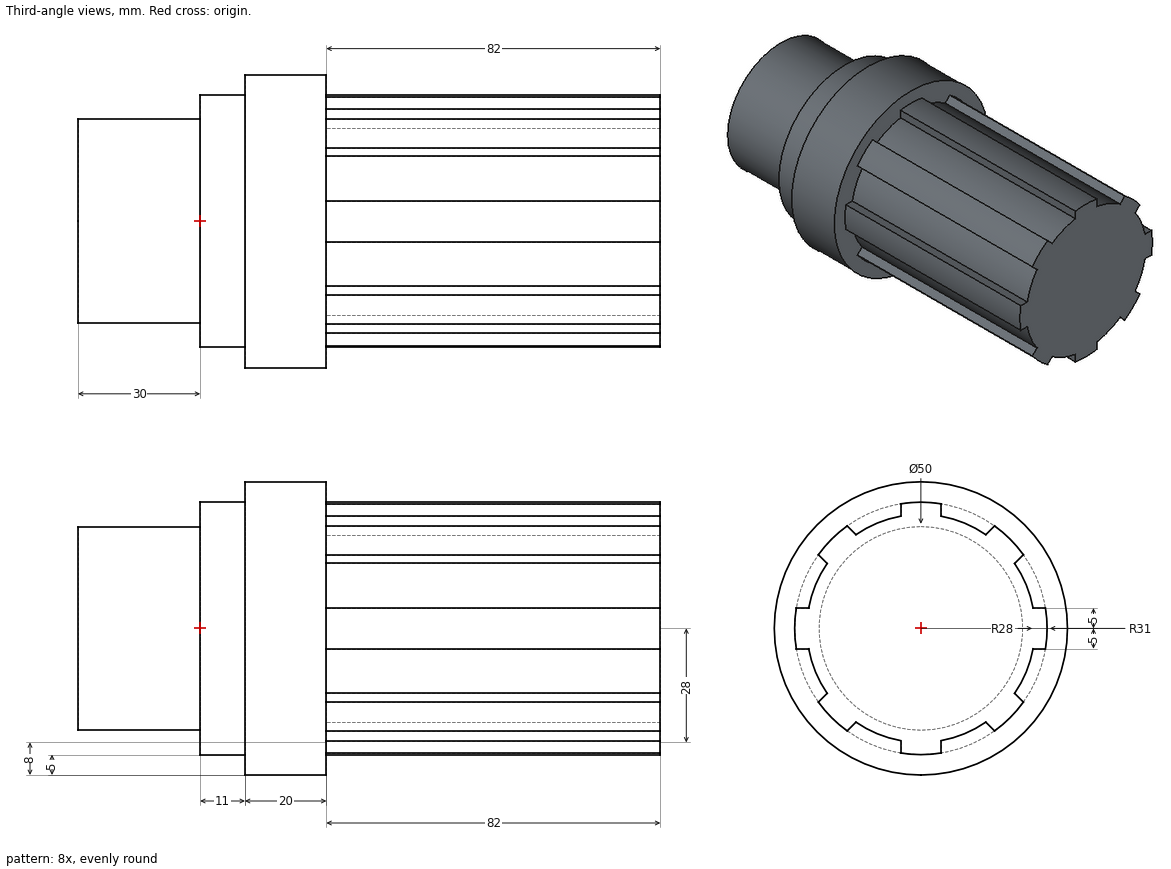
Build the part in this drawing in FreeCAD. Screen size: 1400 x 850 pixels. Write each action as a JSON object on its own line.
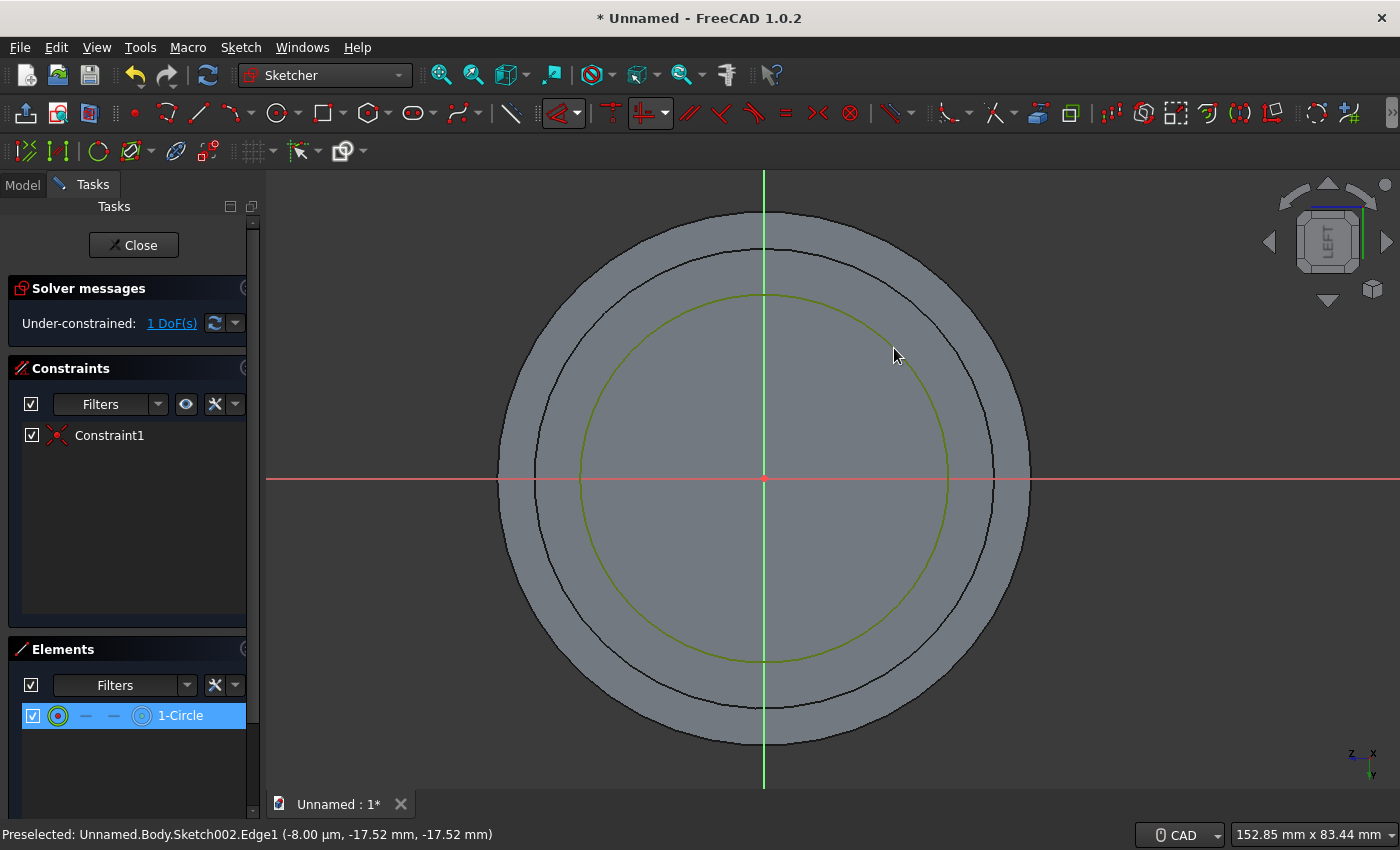
{"action": "key", "text": "k o"}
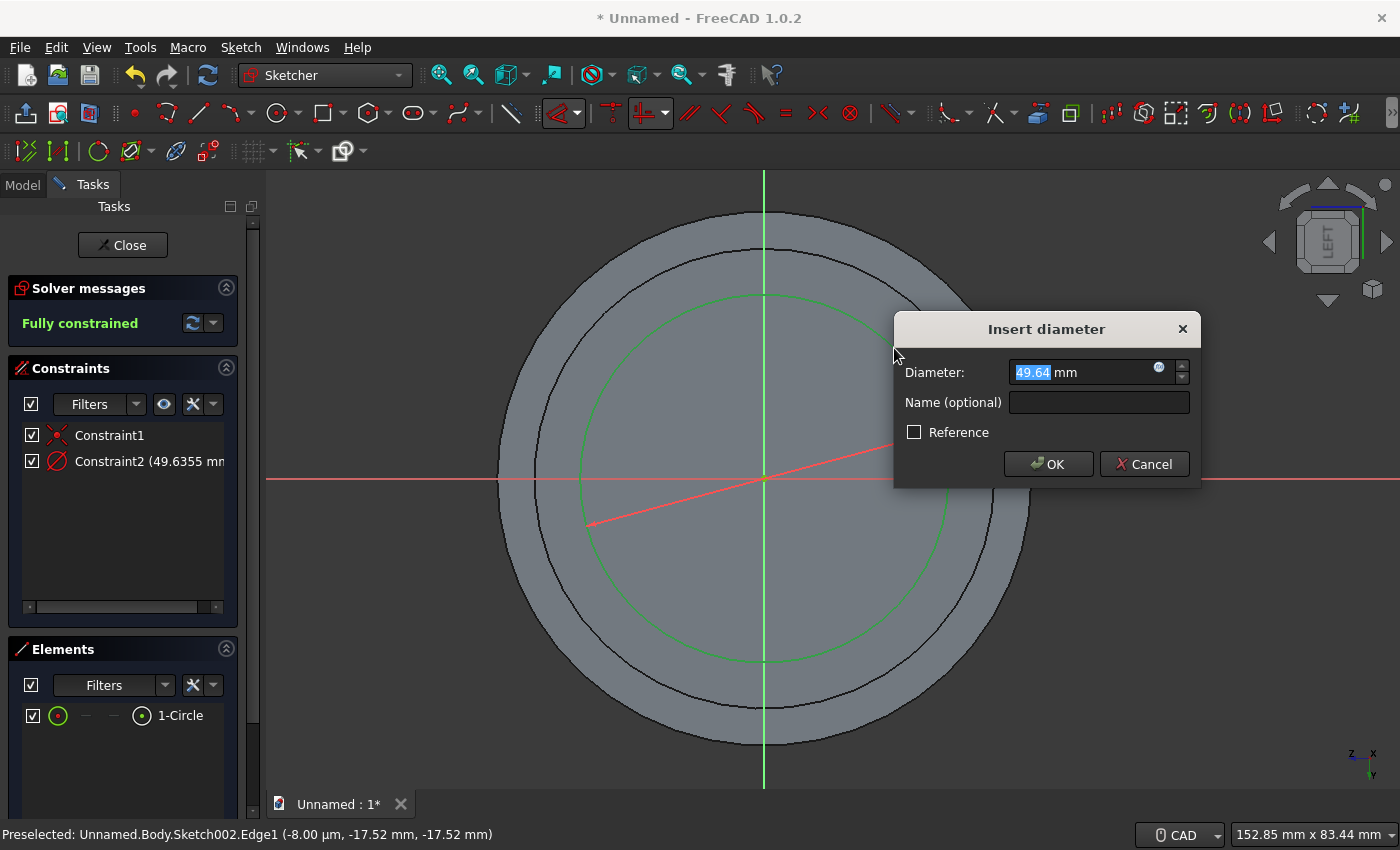
{"action": "type", "text": "50"}
{"action": "key", "text": "Return"}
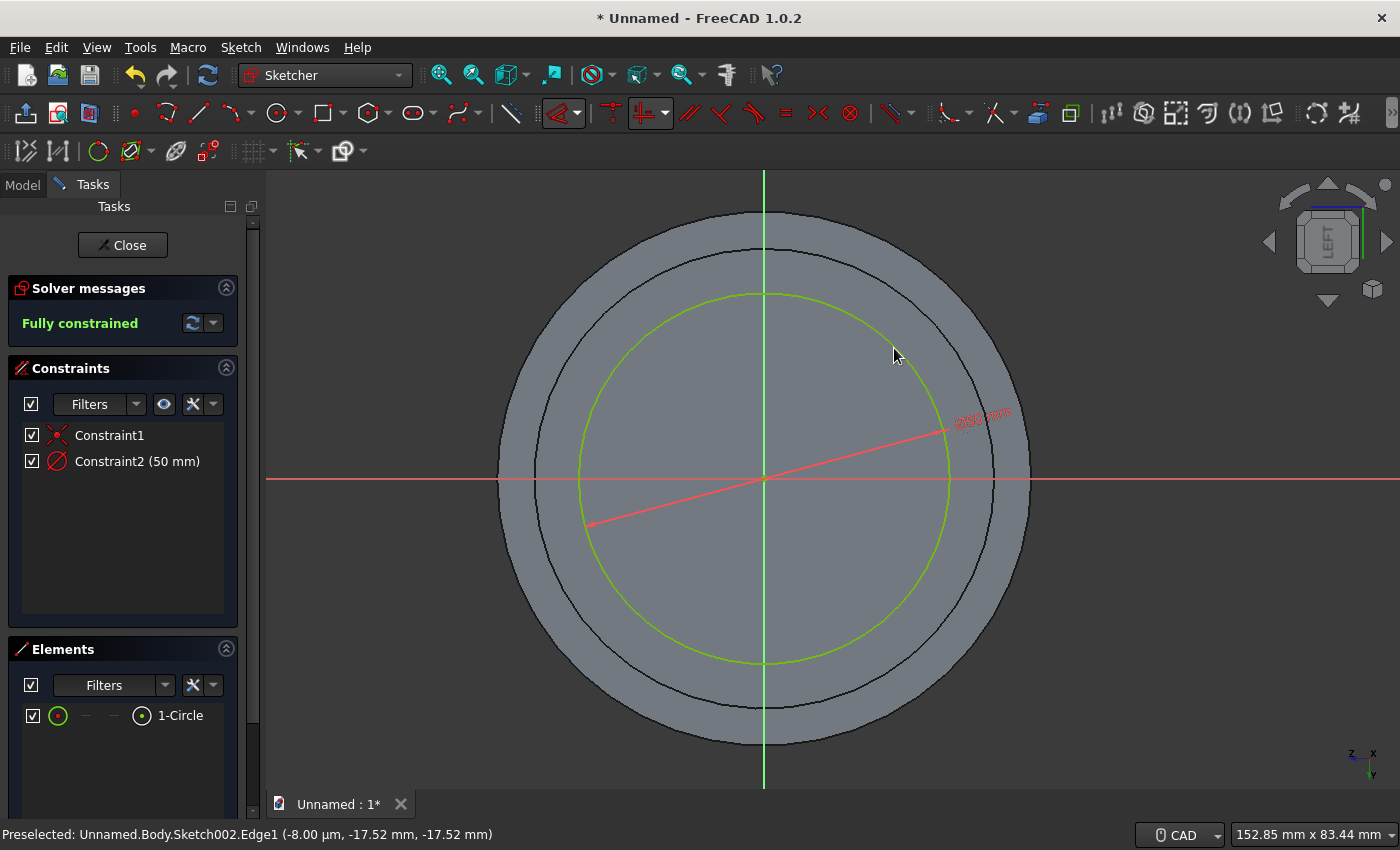
{"action": "left_click", "coordinate": [123, 245]}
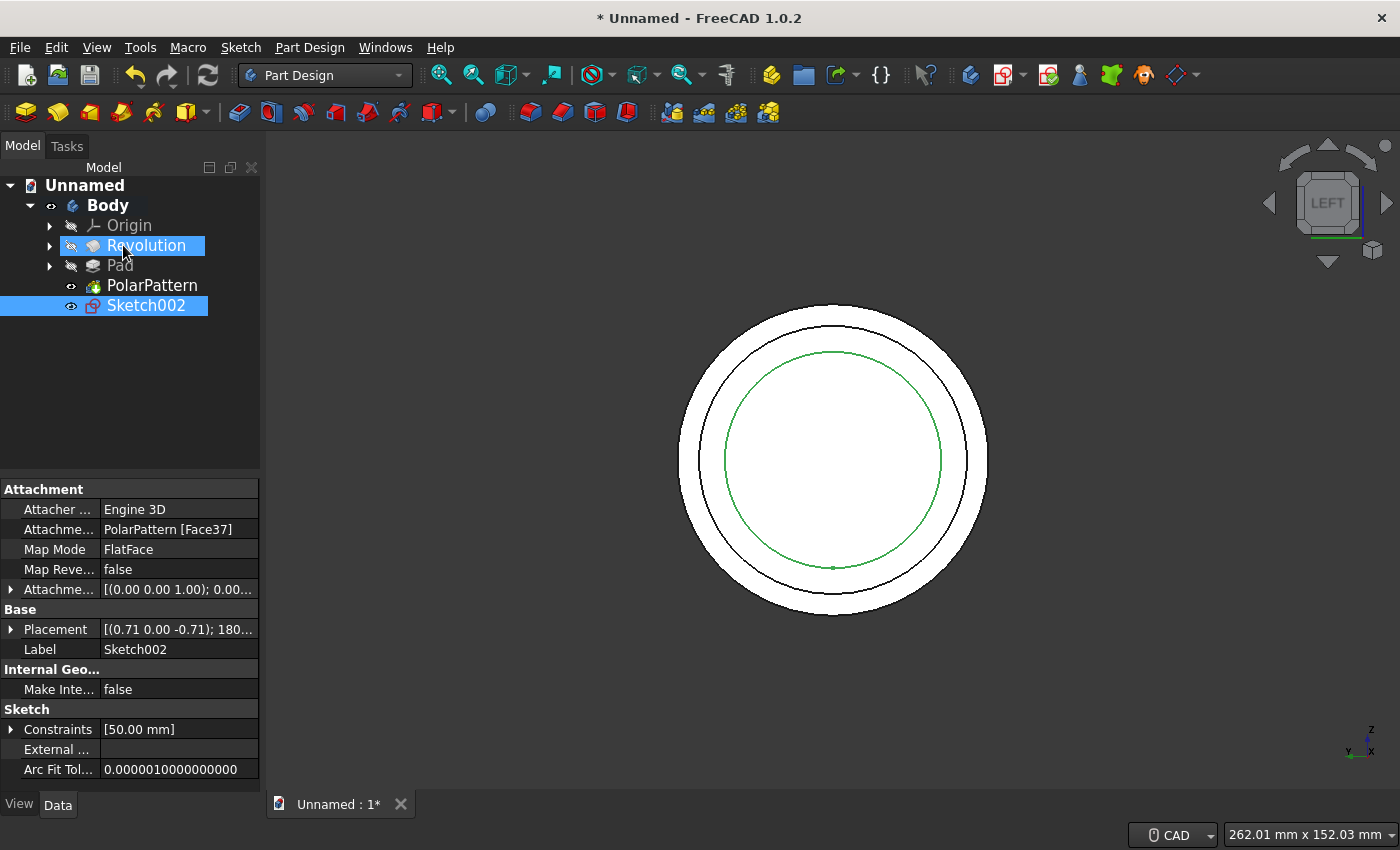
{"action": "left_click", "coordinate": [26, 112]}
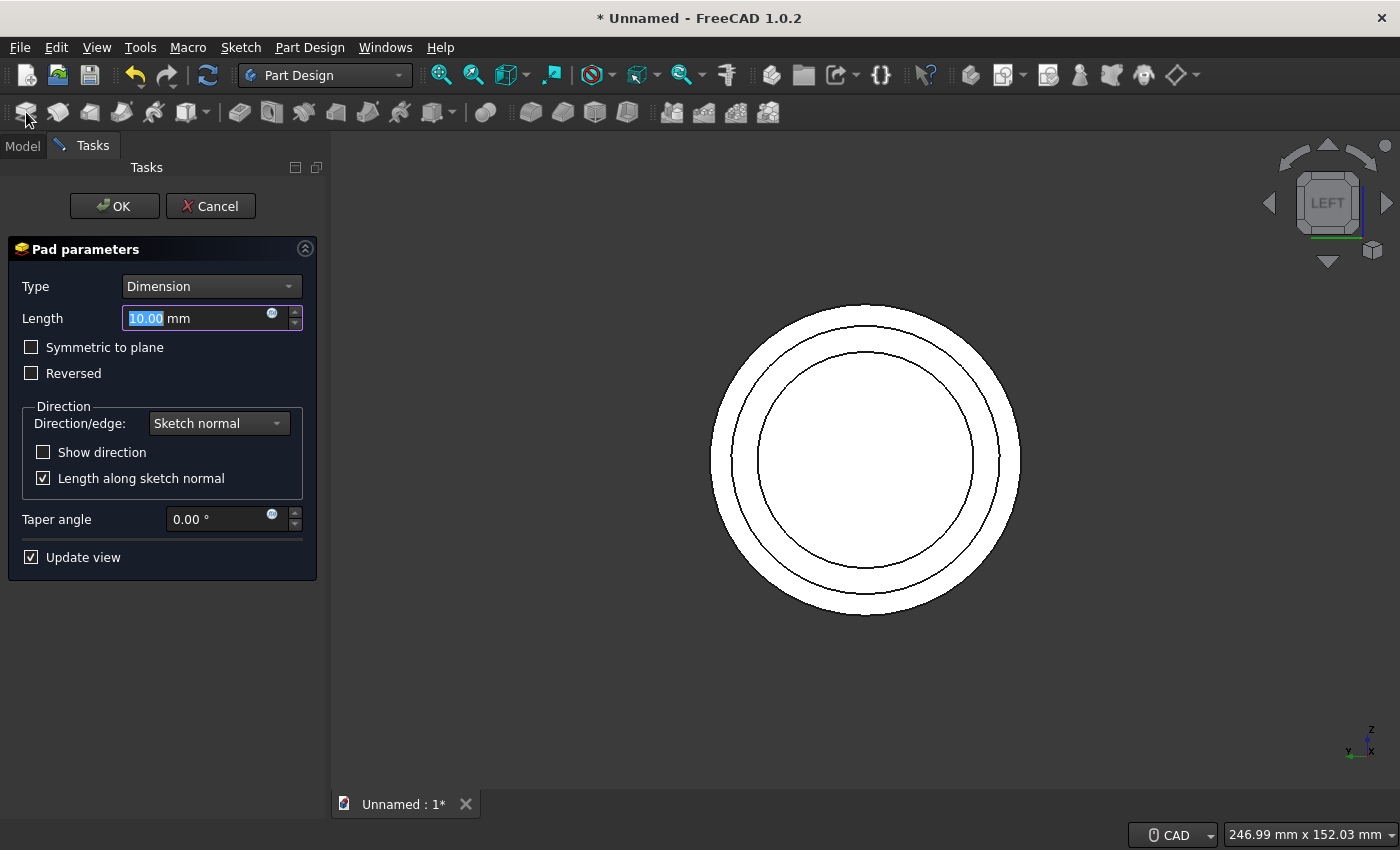
{"action": "type", "text": "30"}
{"action": "key", "text": "Tab"}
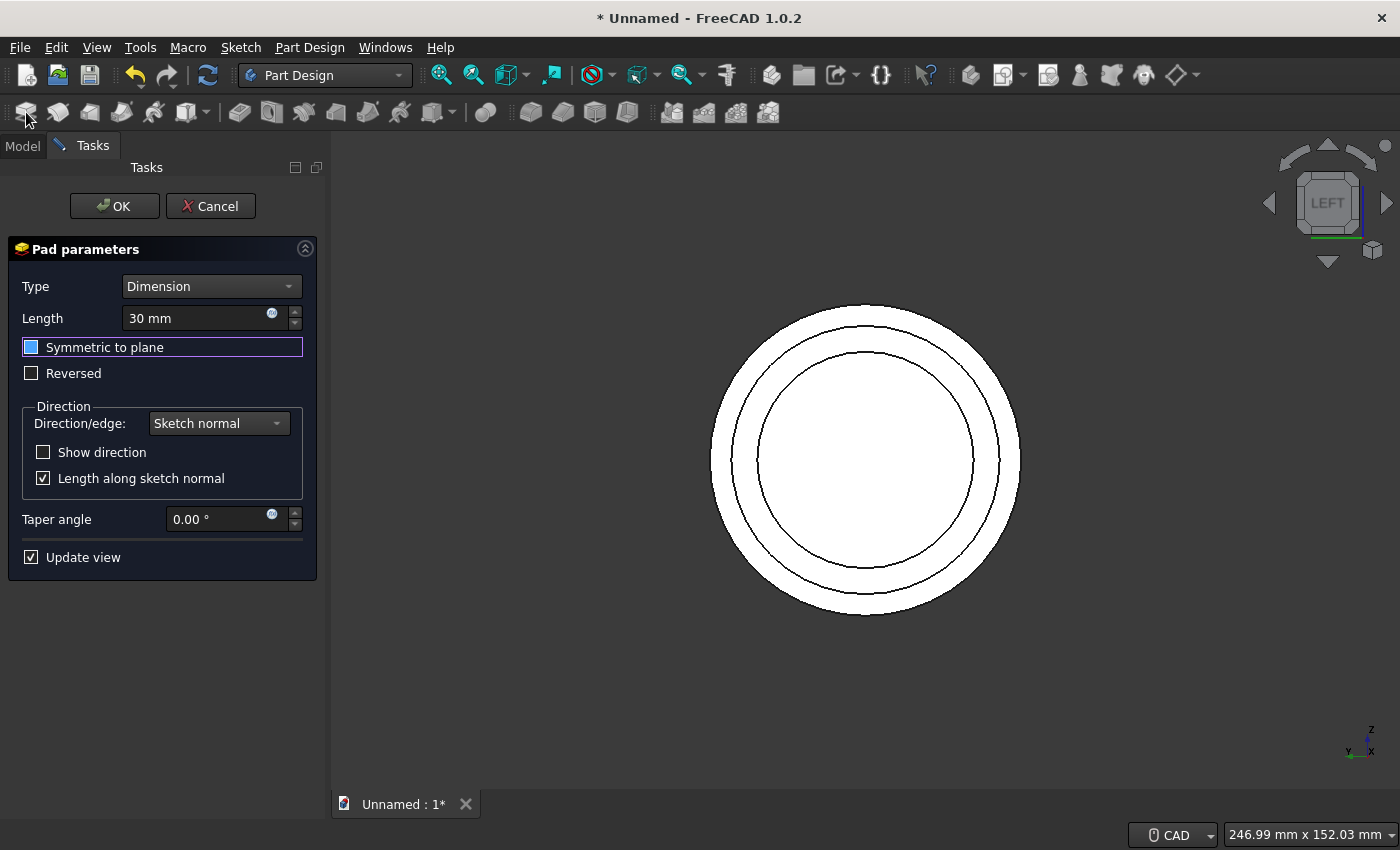
{"action": "left_click", "coordinate": [115, 206]}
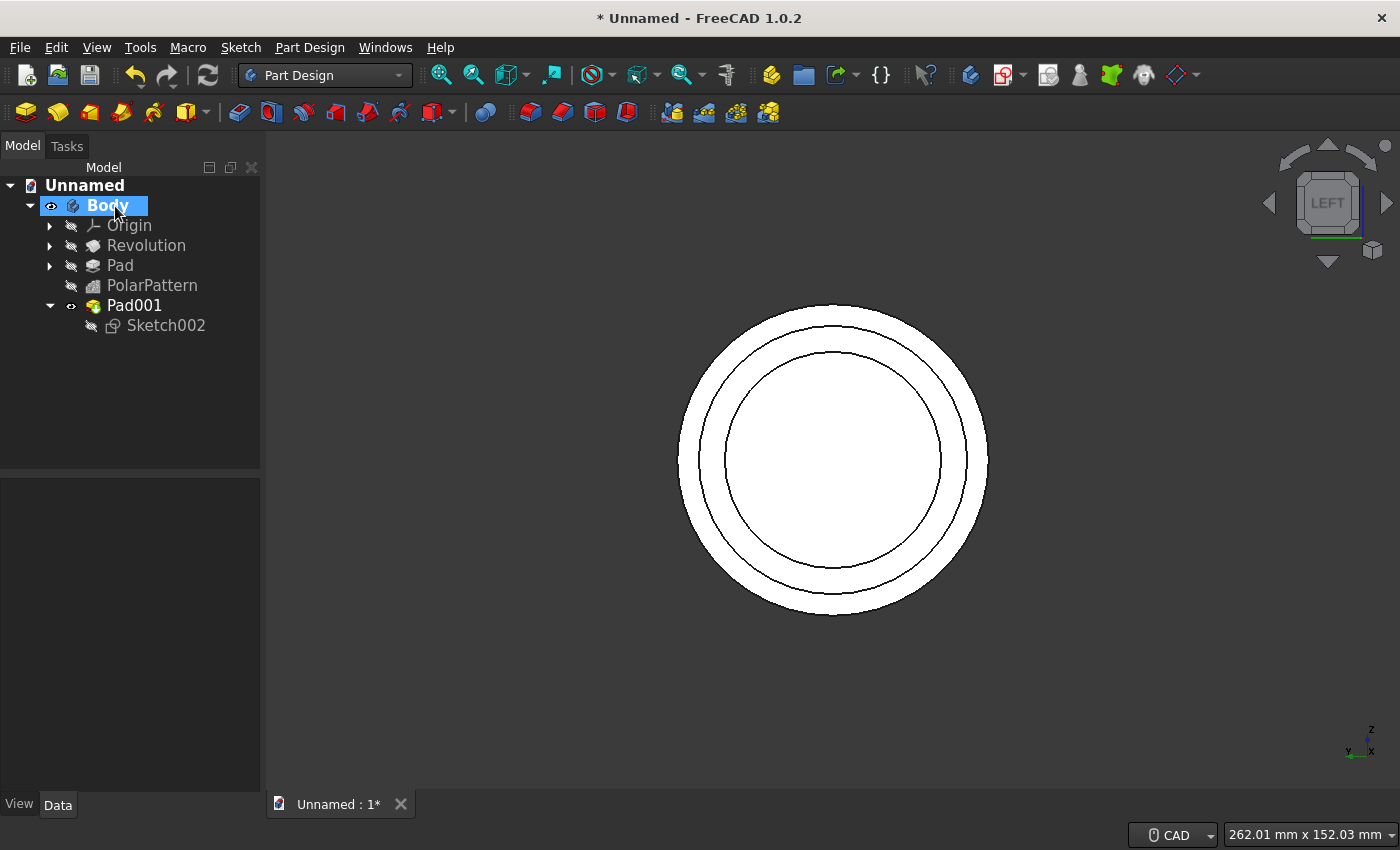
{"action": "key", "text": "0"}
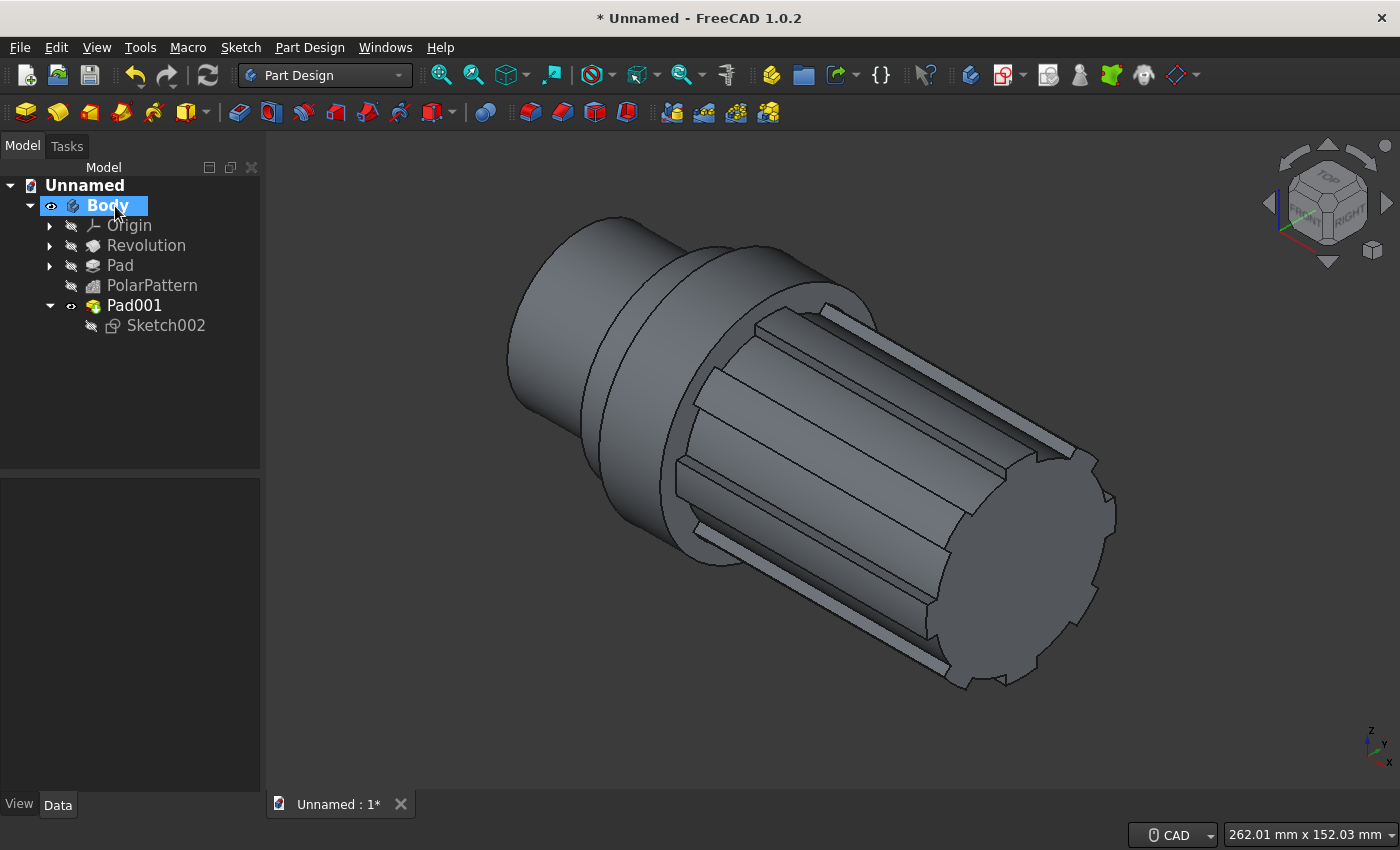
{"action": "left_click", "coordinate": [442, 76]}